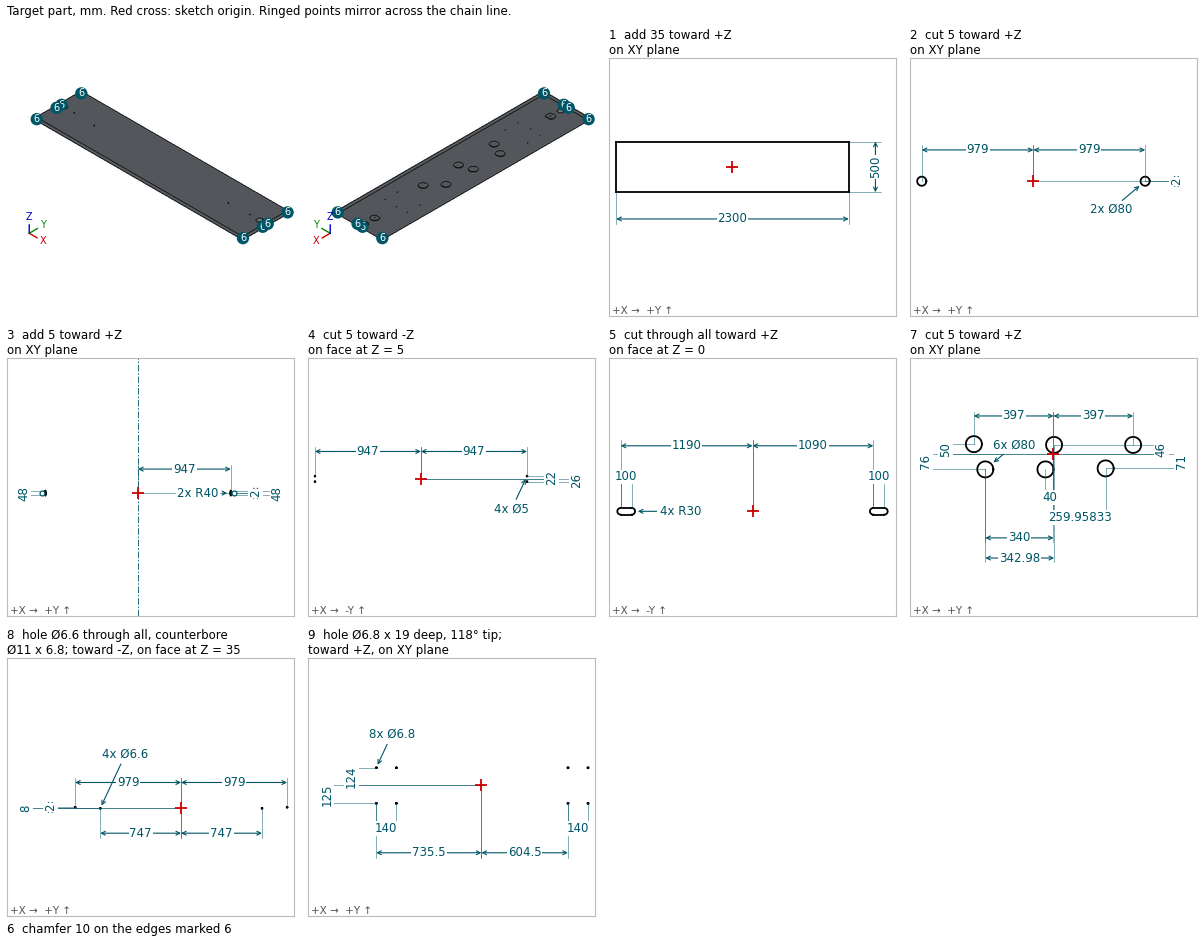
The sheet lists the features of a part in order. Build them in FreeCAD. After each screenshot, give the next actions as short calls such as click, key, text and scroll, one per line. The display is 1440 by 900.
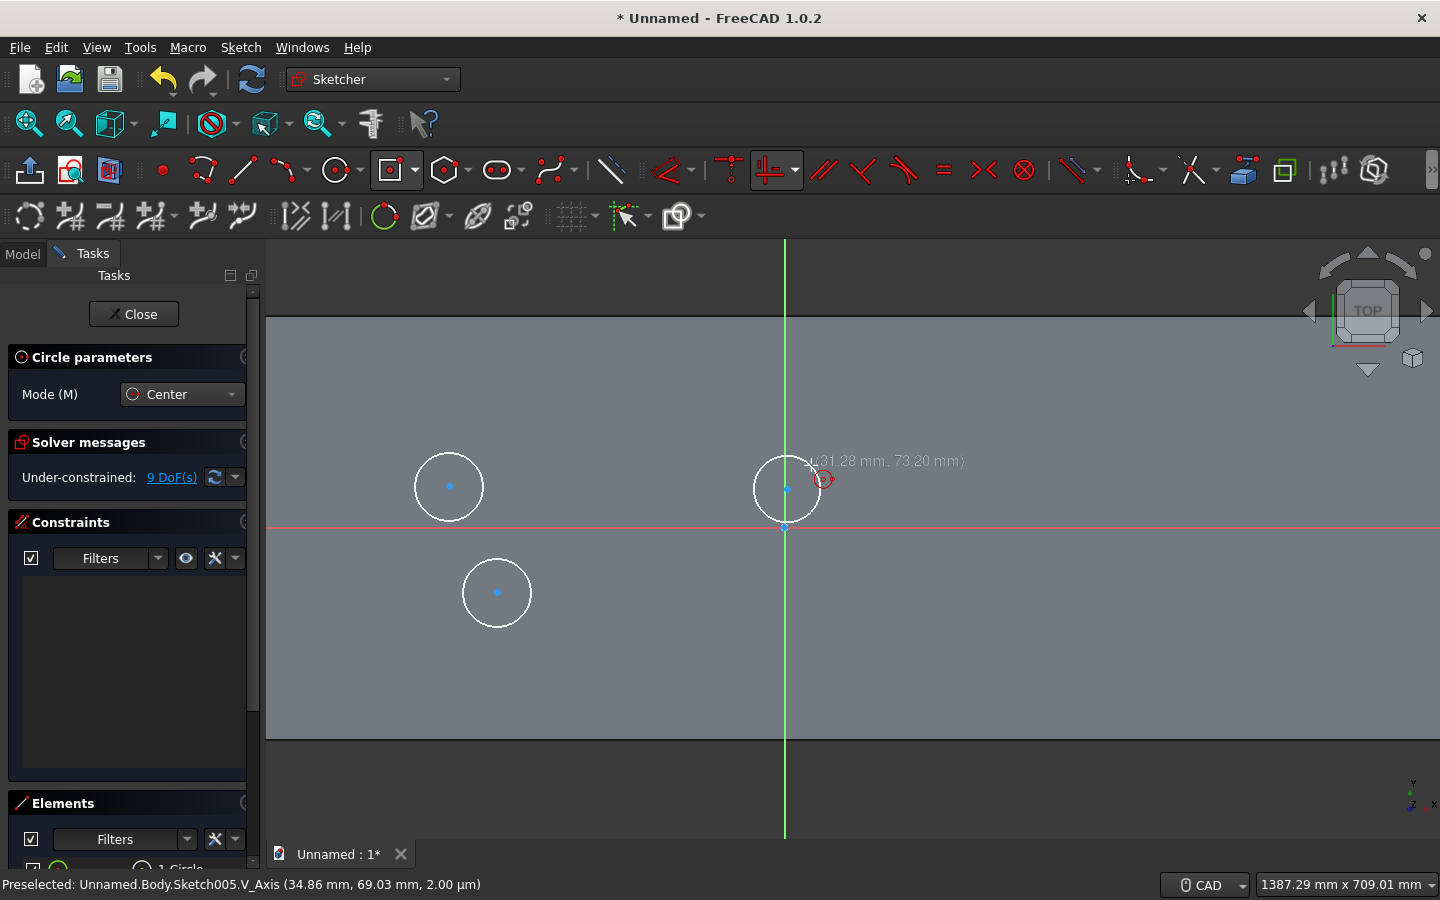
click(751, 592)
click(727, 568)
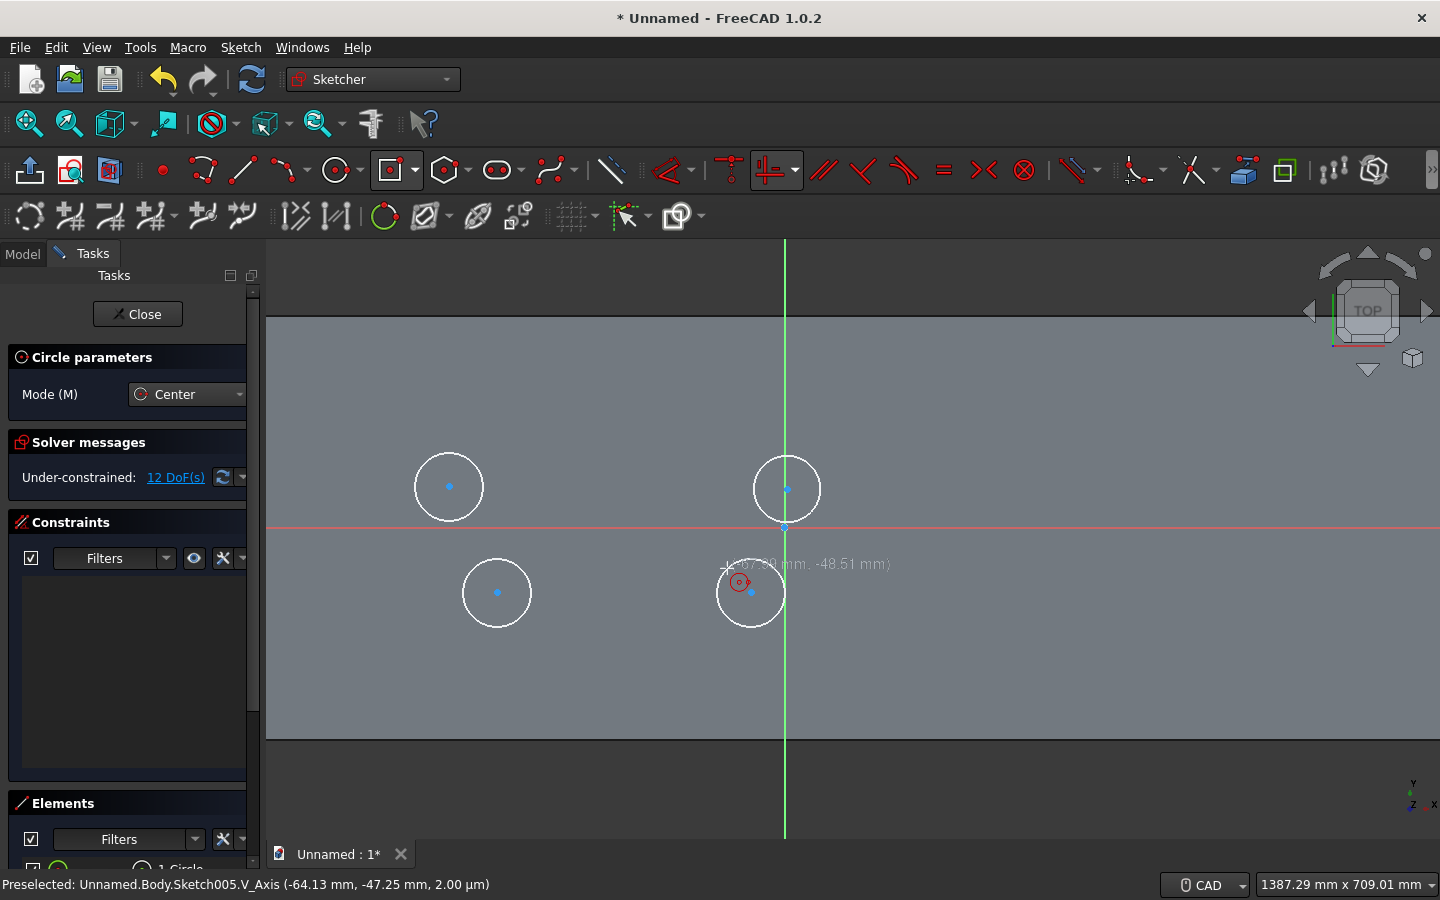
click(1005, 588)
click(1028, 564)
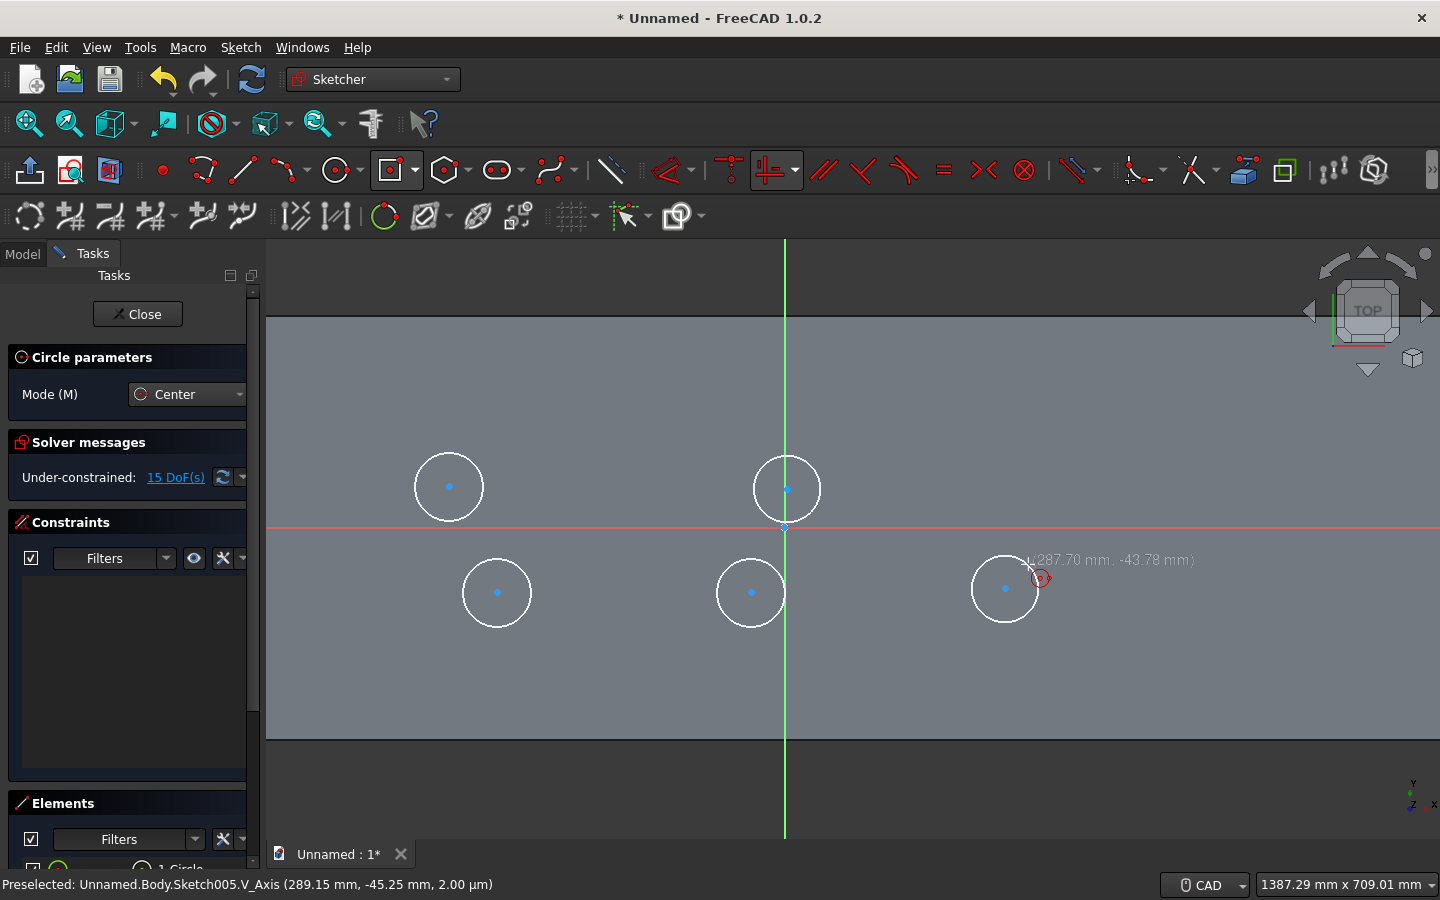
click(1120, 489)
click(1144, 465)
key(Escape)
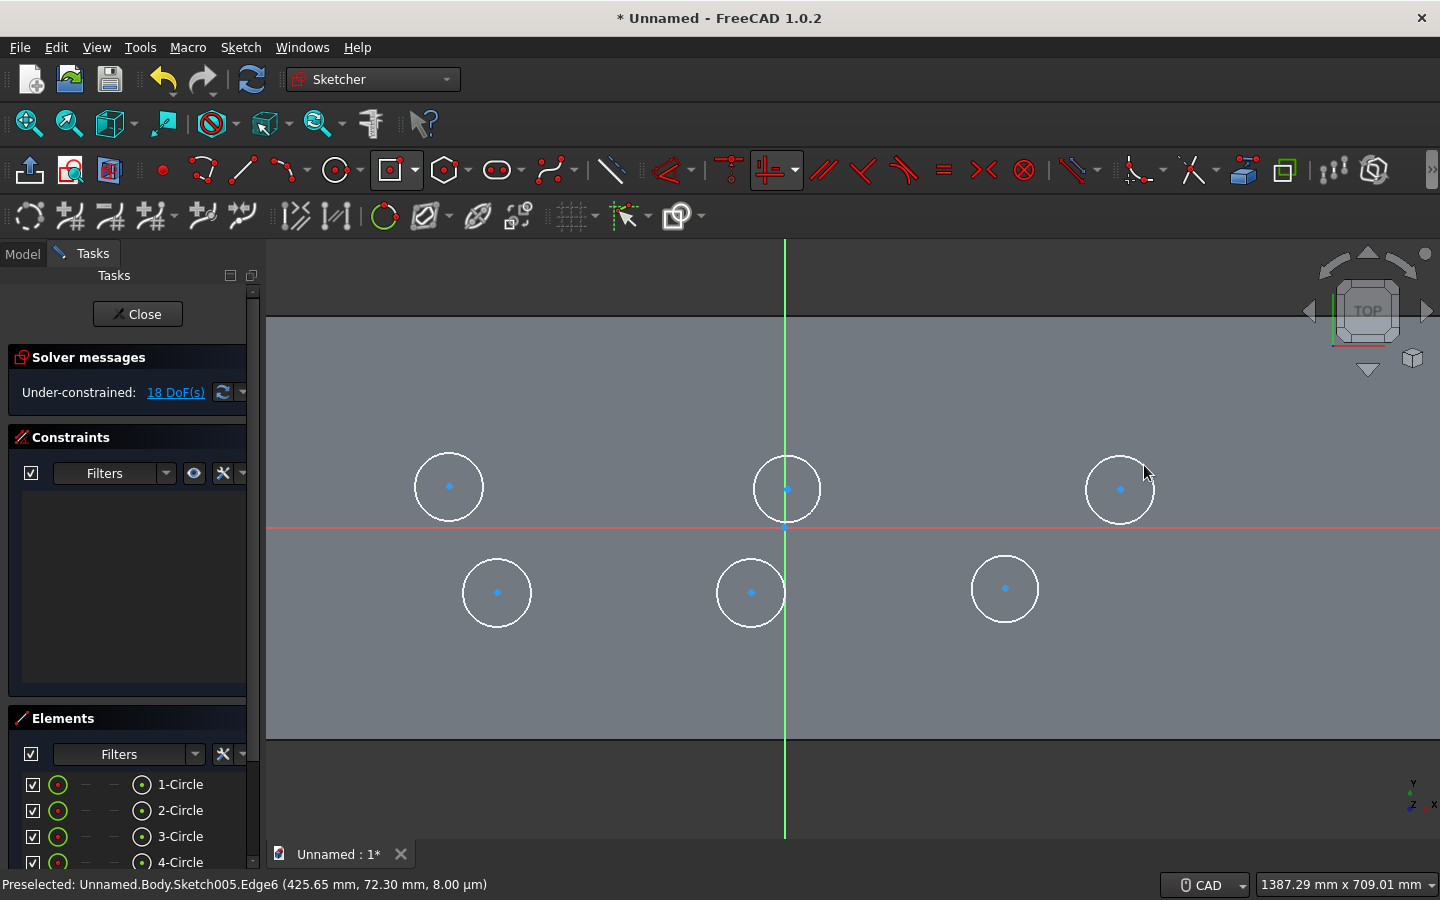
click(521, 569)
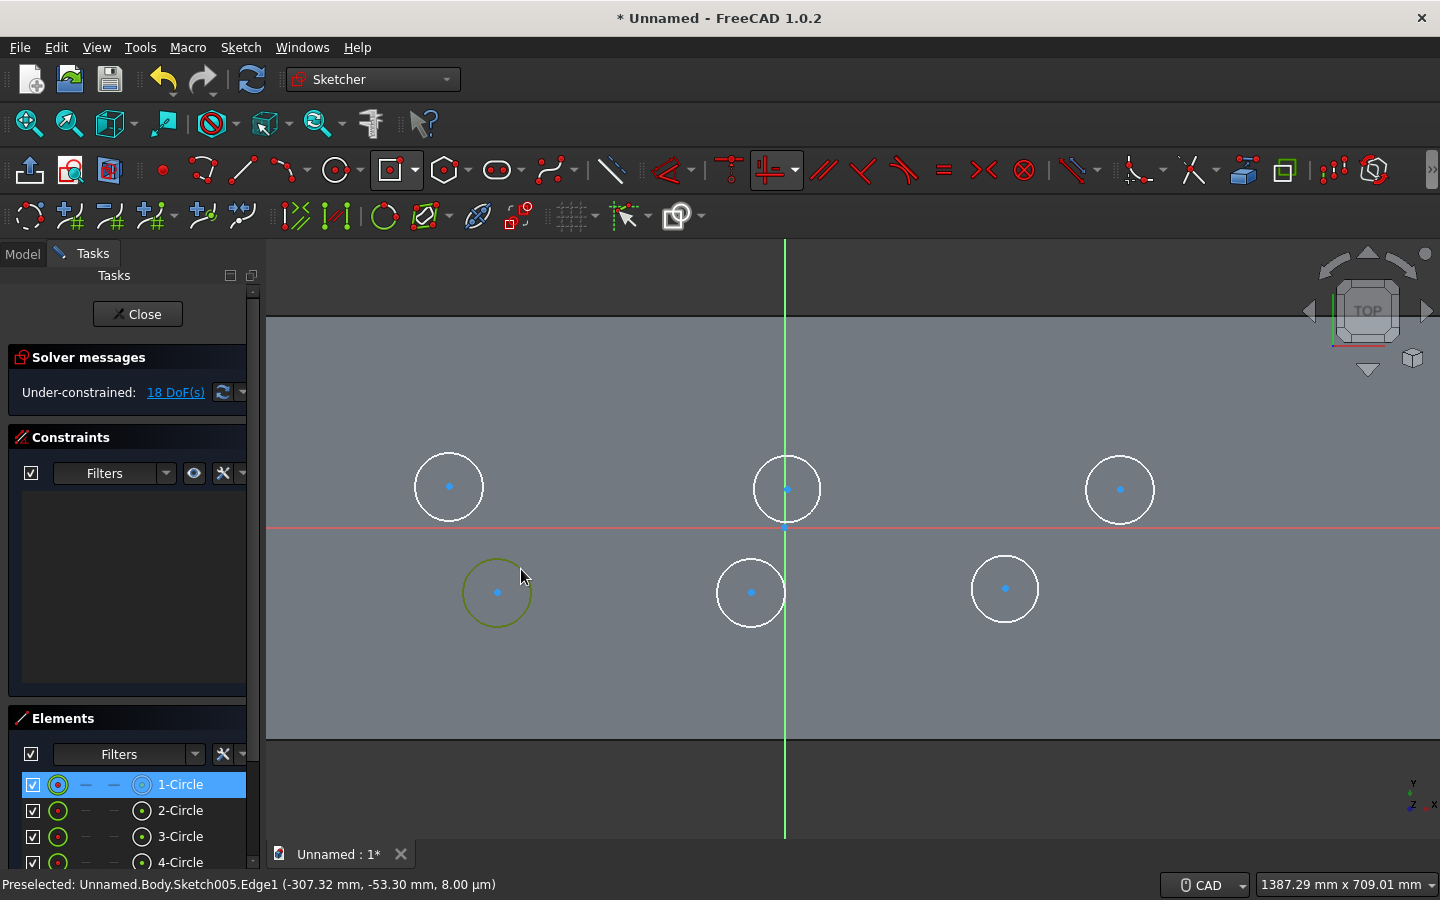
click(473, 463)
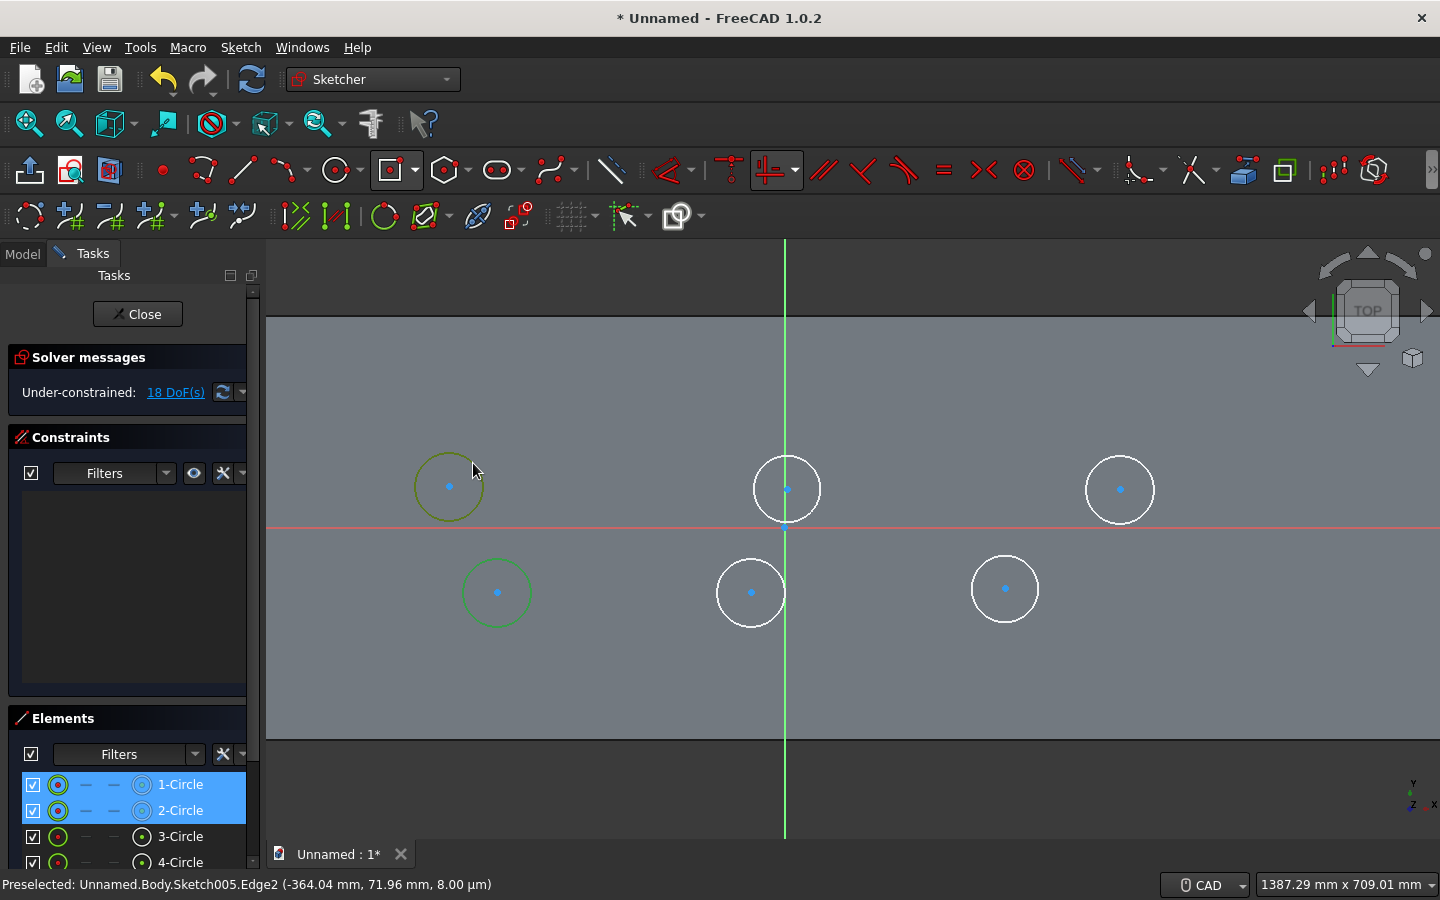
click(811, 466)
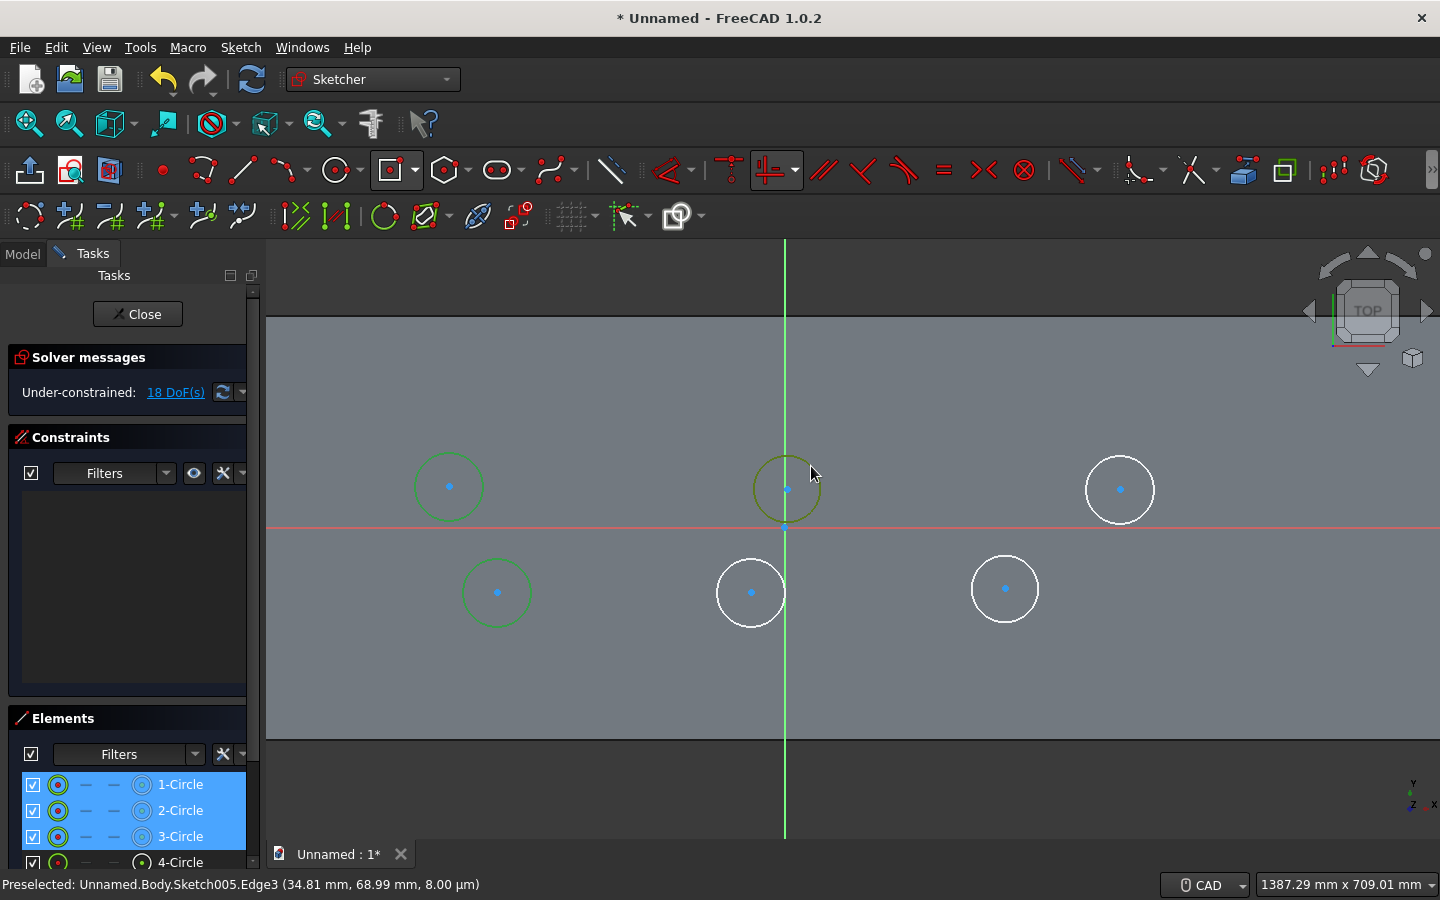
scroll(775, 569, up, 2)